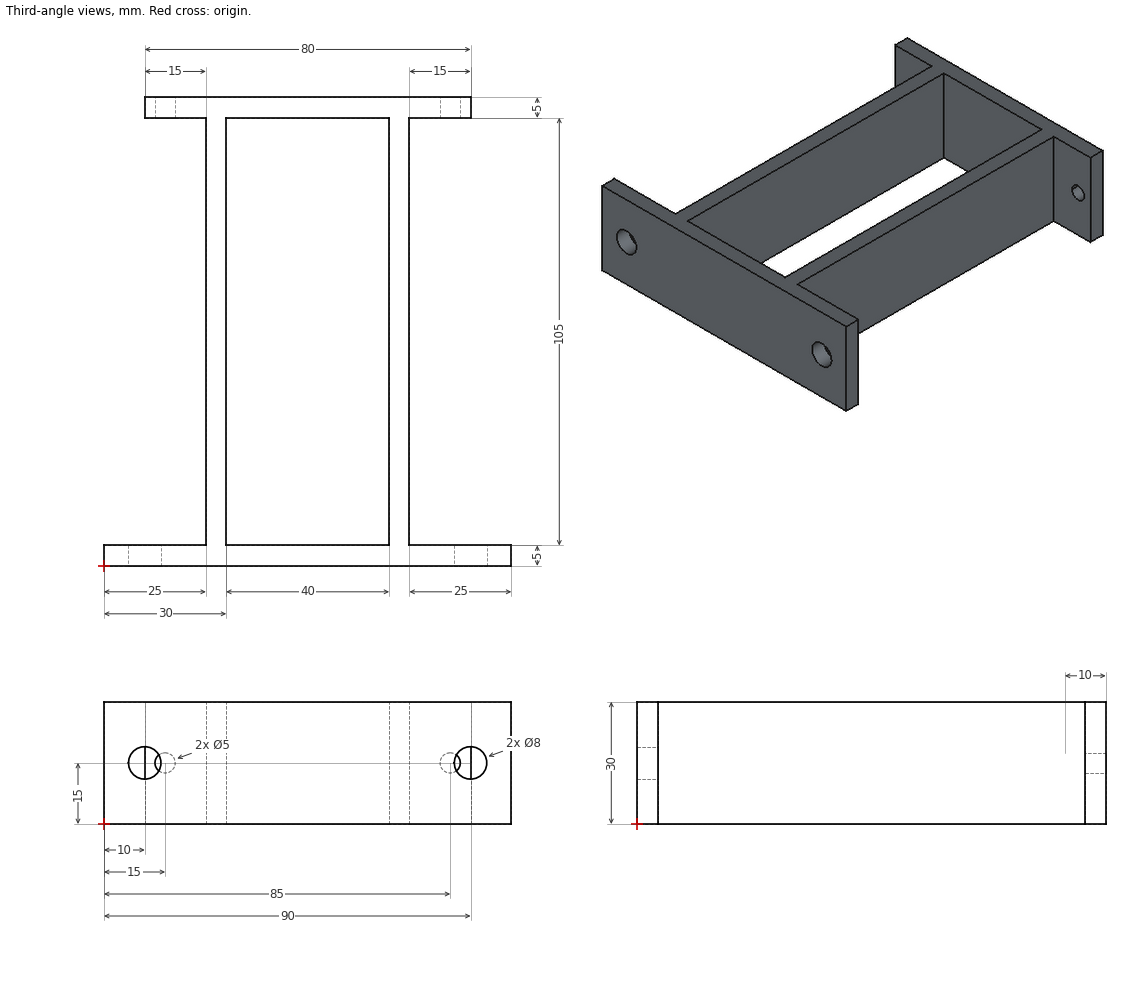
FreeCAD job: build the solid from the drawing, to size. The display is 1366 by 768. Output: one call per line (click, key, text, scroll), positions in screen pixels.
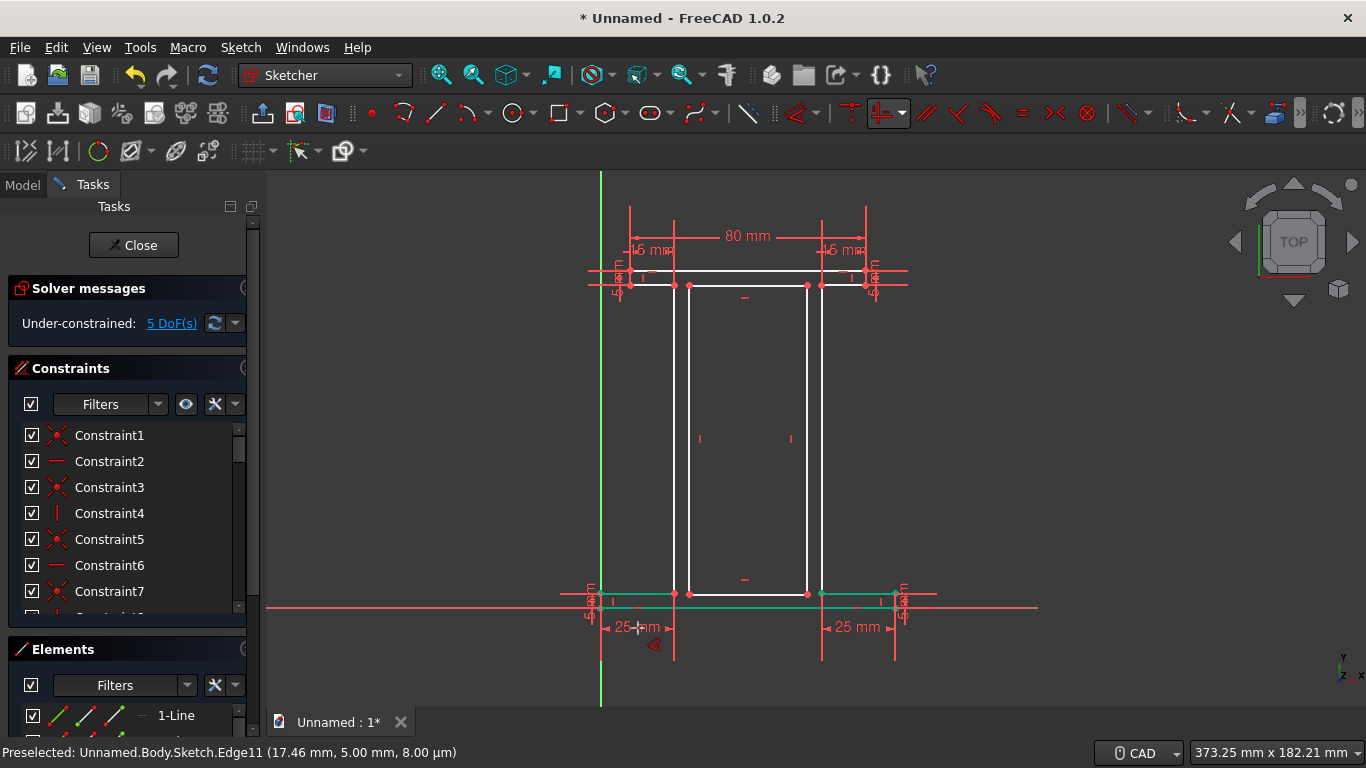
click(724, 595)
click(748, 629)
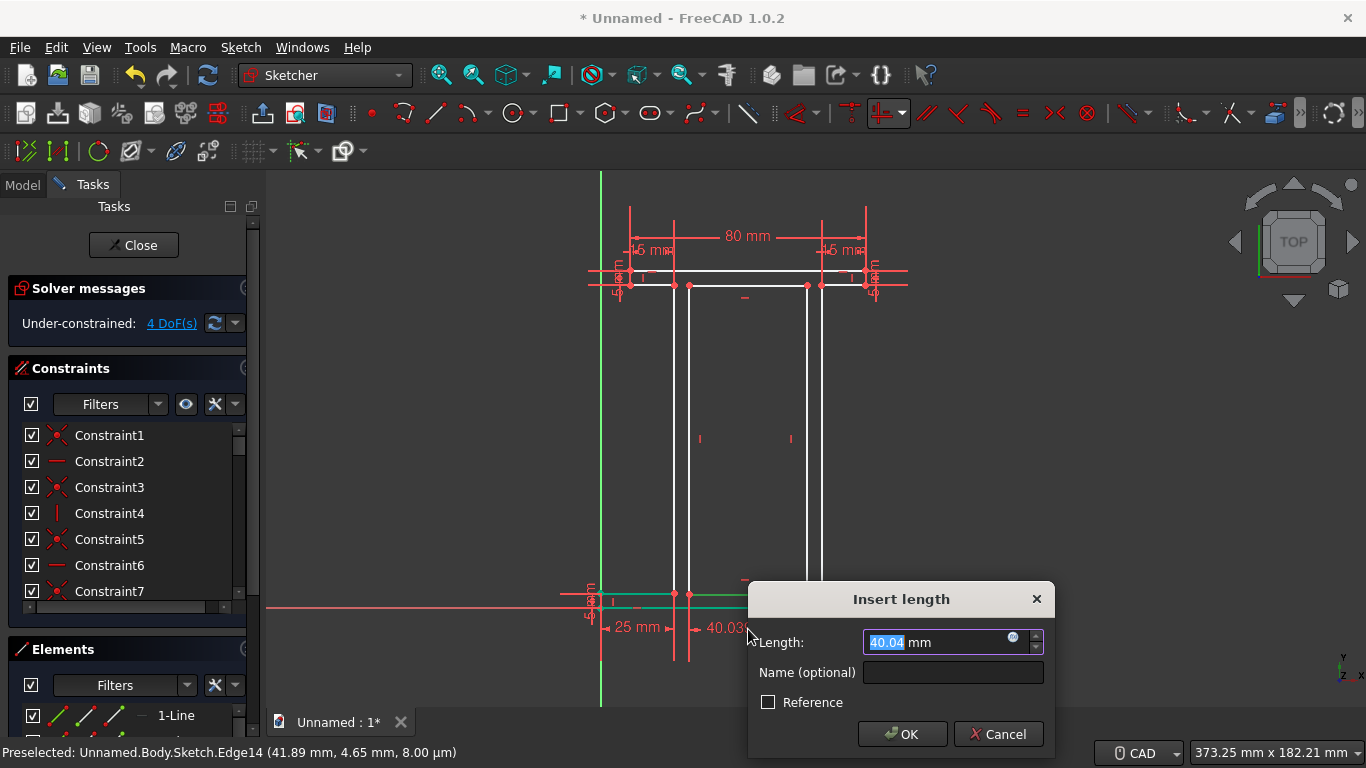
text(40)
key(Return)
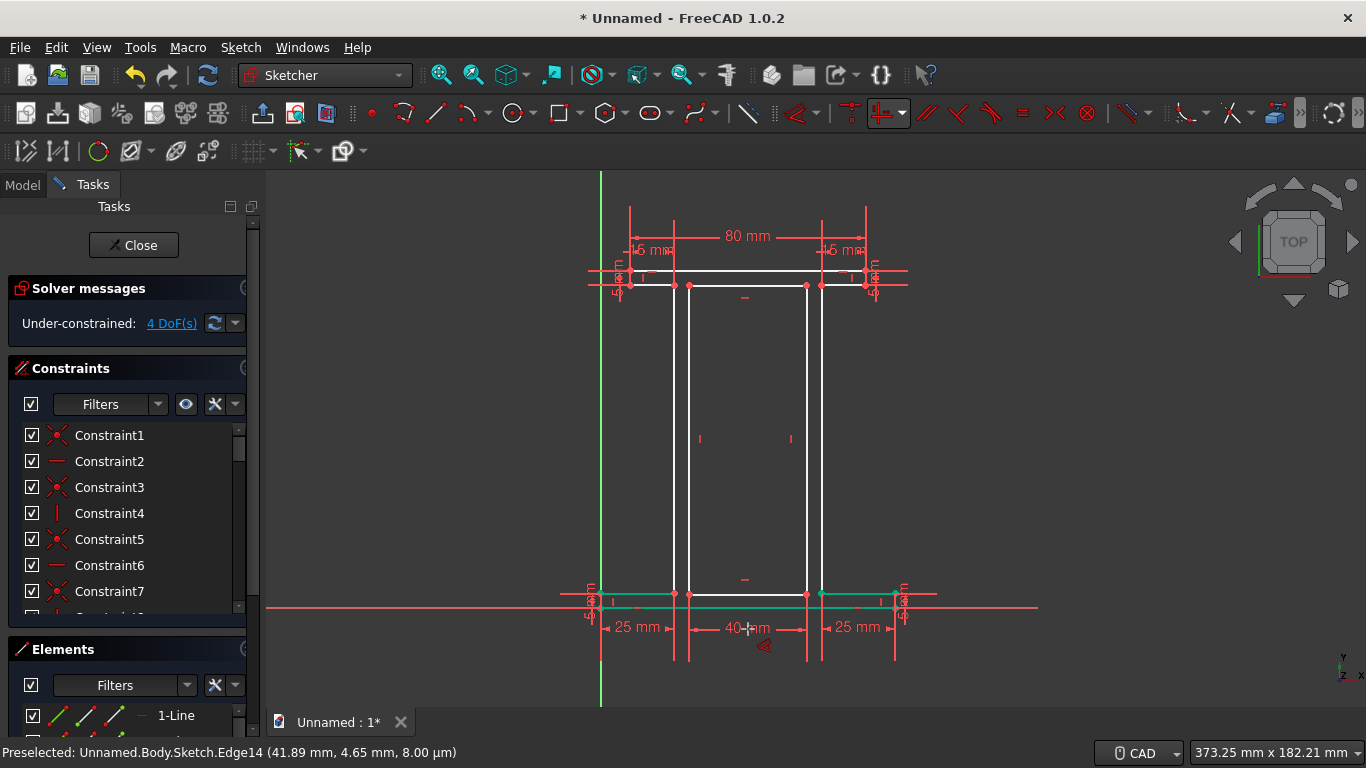
scroll(689, 595, up, 5)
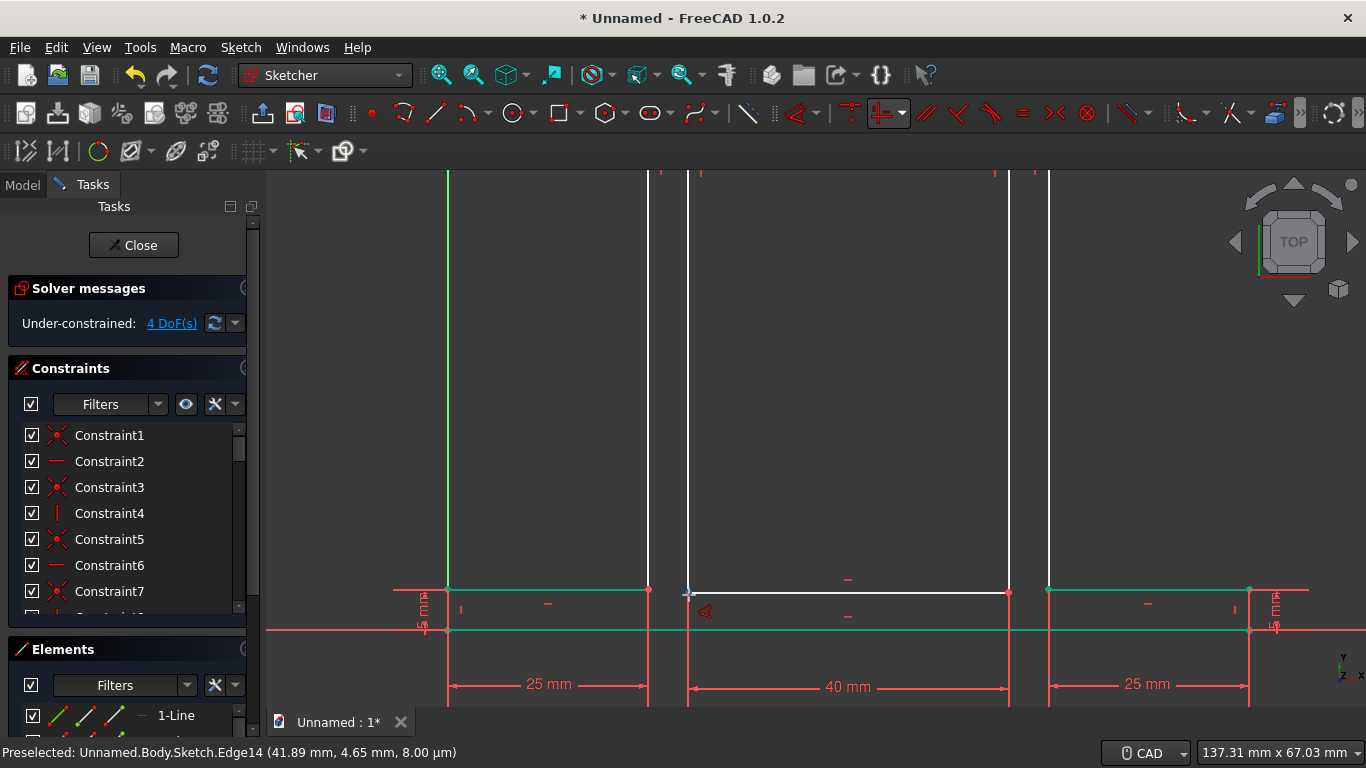
click(688, 593)
click(722, 611)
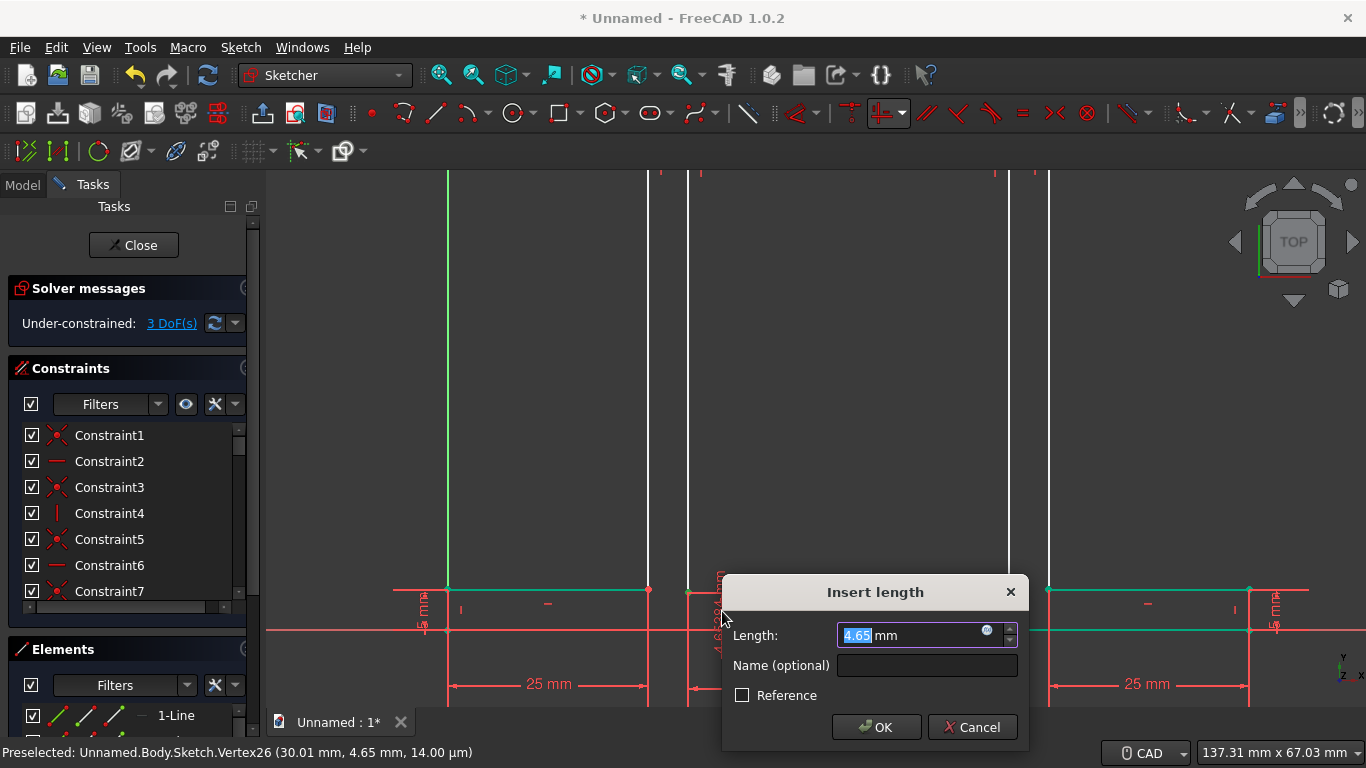
text(5)
key(Return)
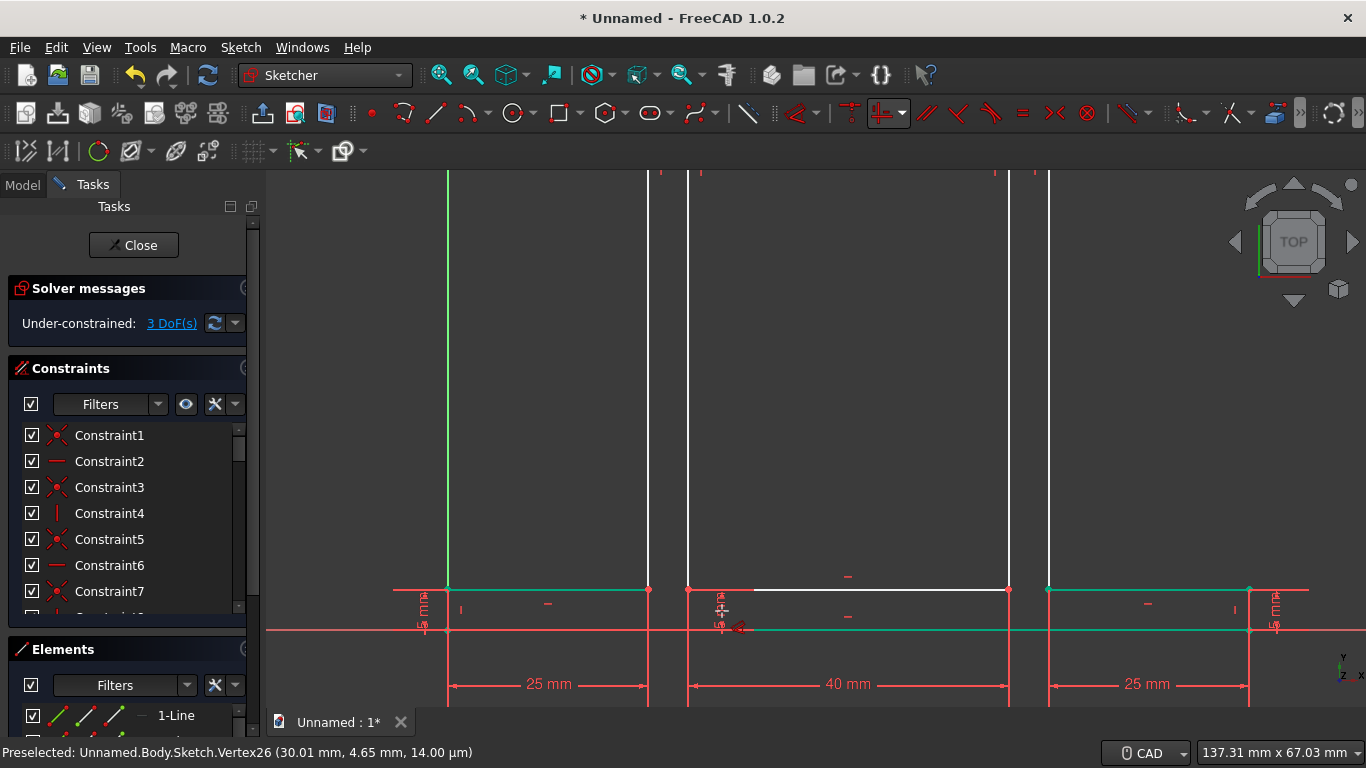
click(1049, 338)
click(1083, 394)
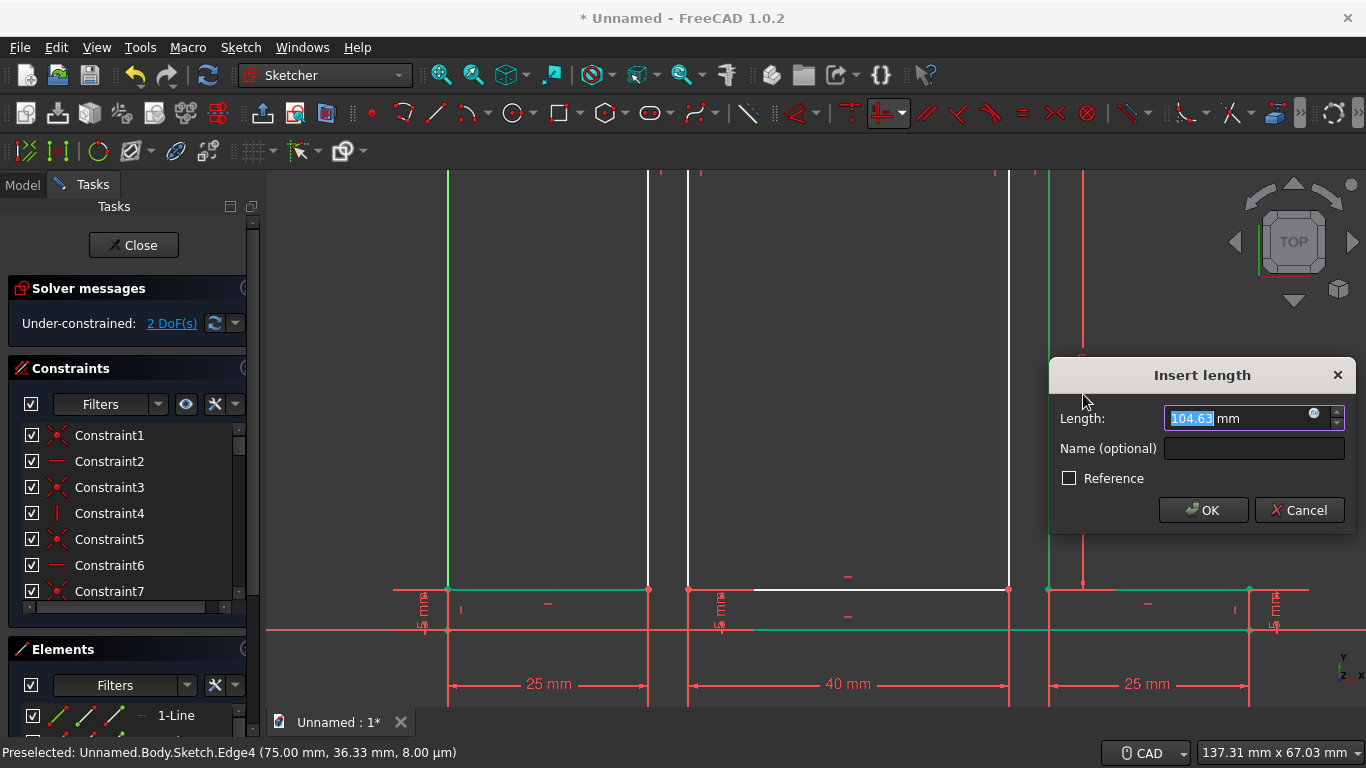
text(105)
key(Return)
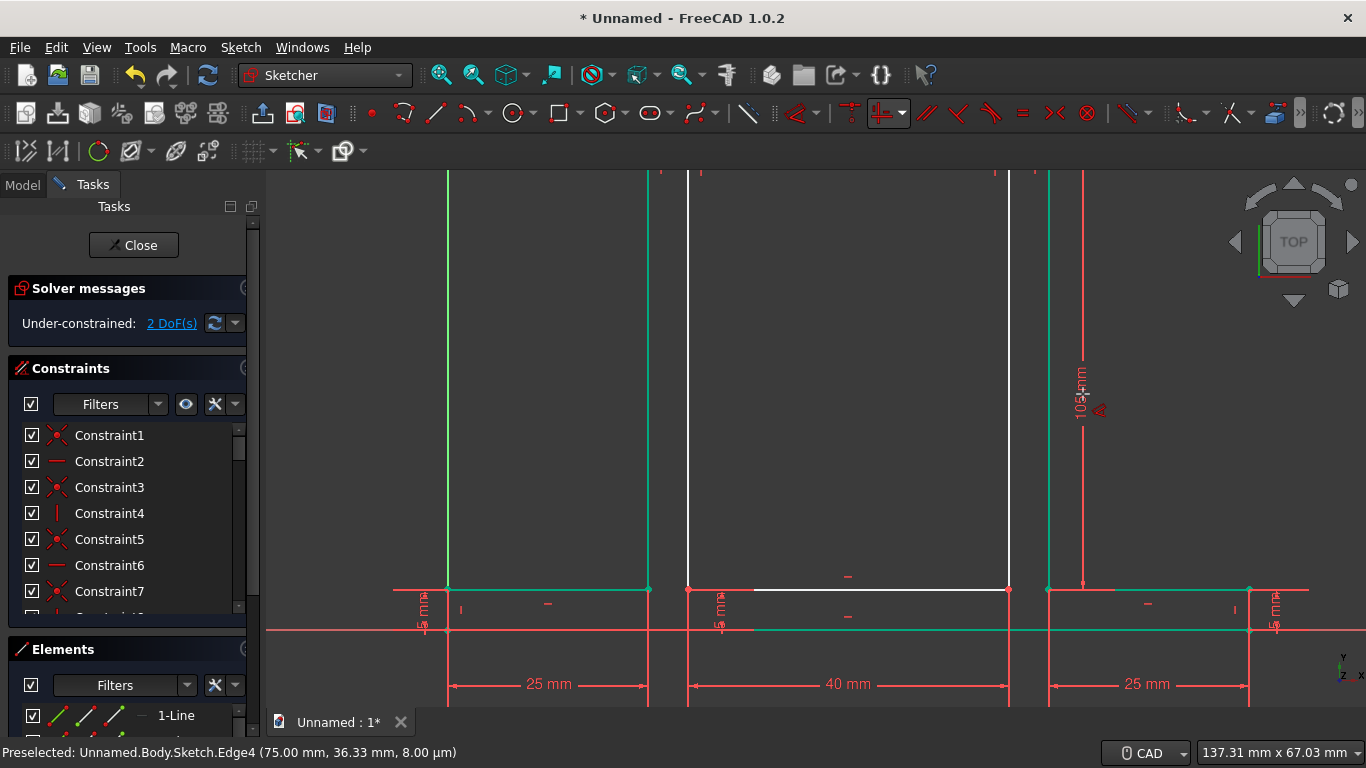
click(688, 339)
click(722, 394)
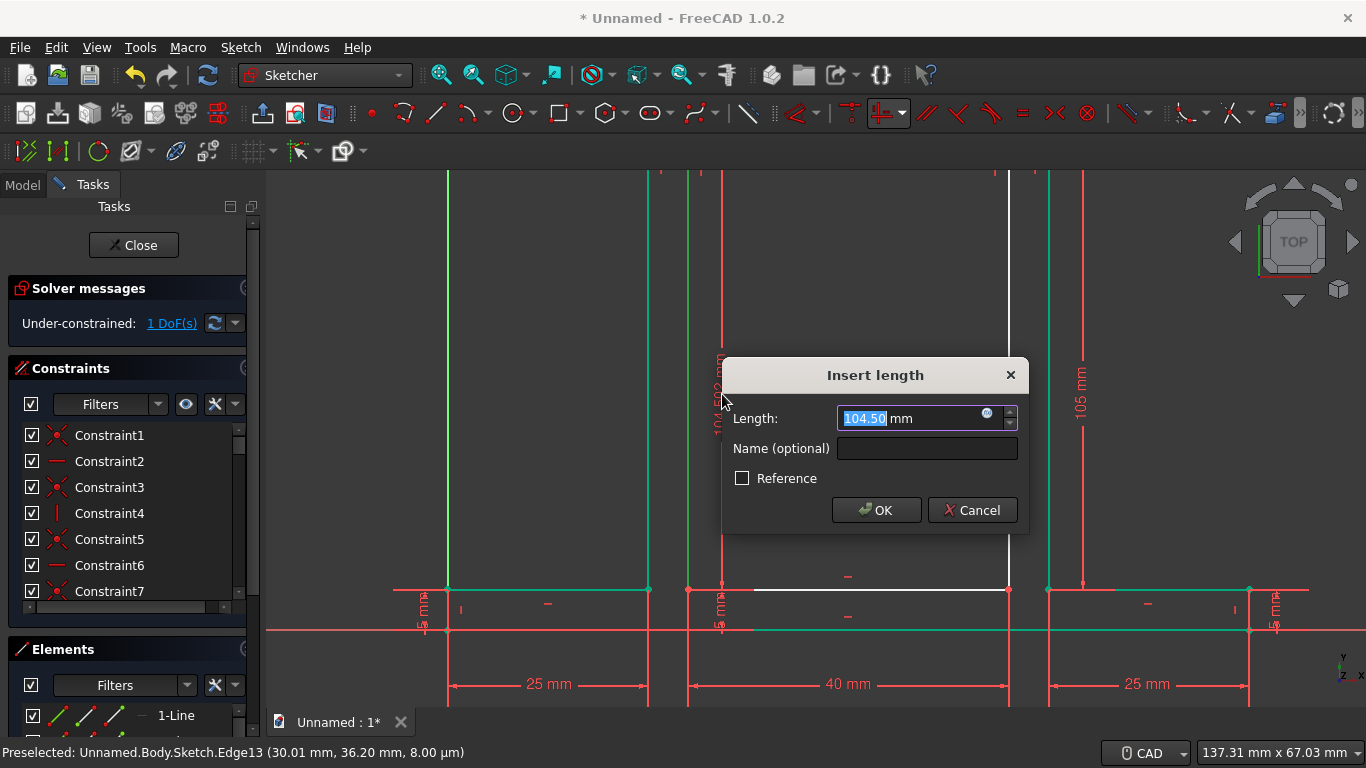
text(105)
key(Return)